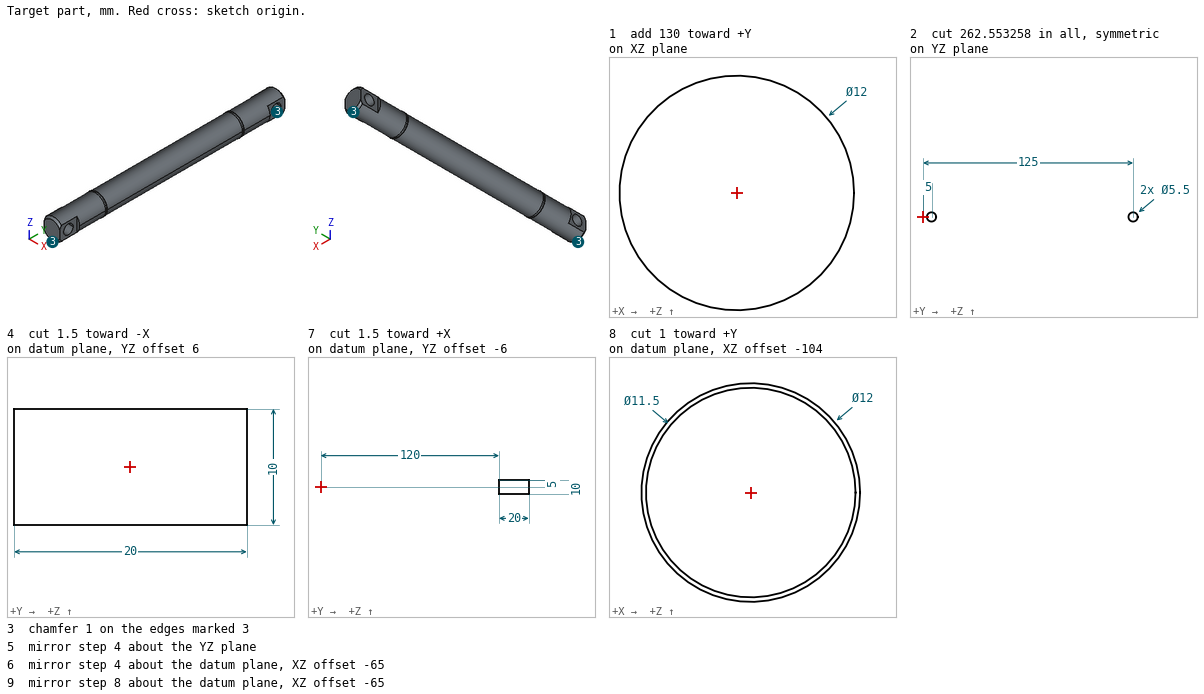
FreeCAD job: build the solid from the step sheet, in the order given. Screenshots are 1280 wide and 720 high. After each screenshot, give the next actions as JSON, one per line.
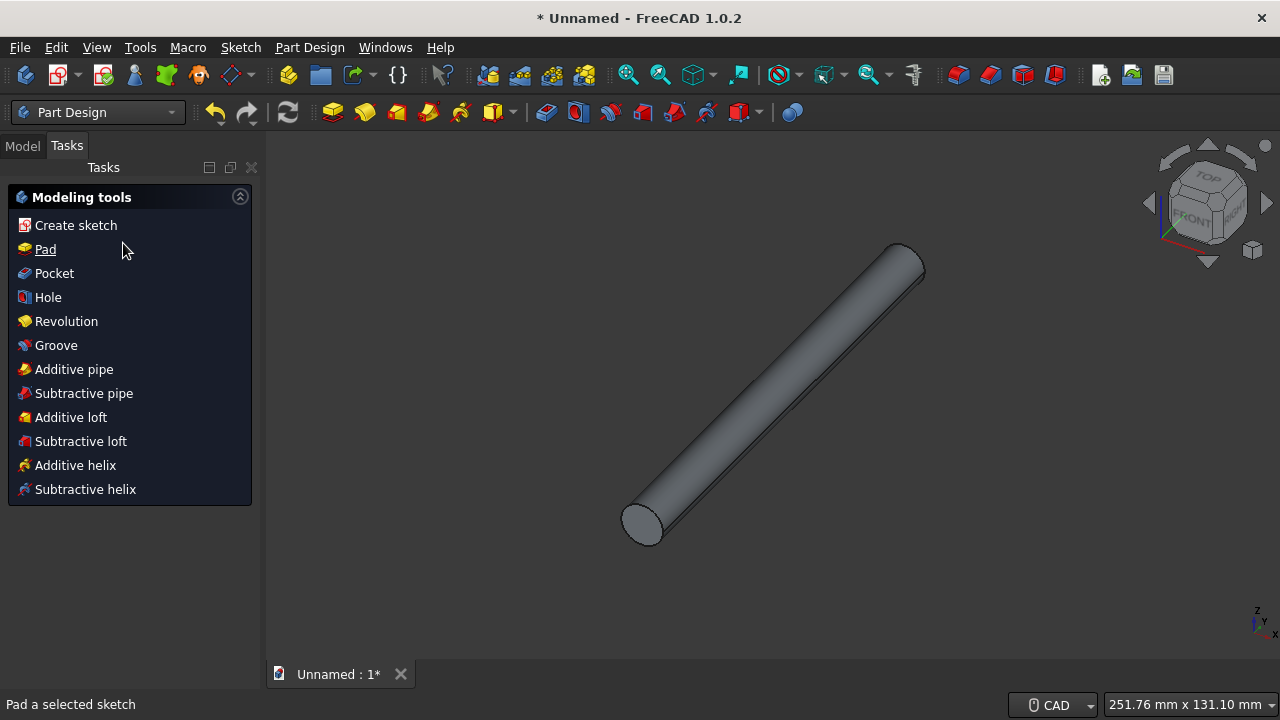
{"action": "left_click", "coordinate": [548, 112]}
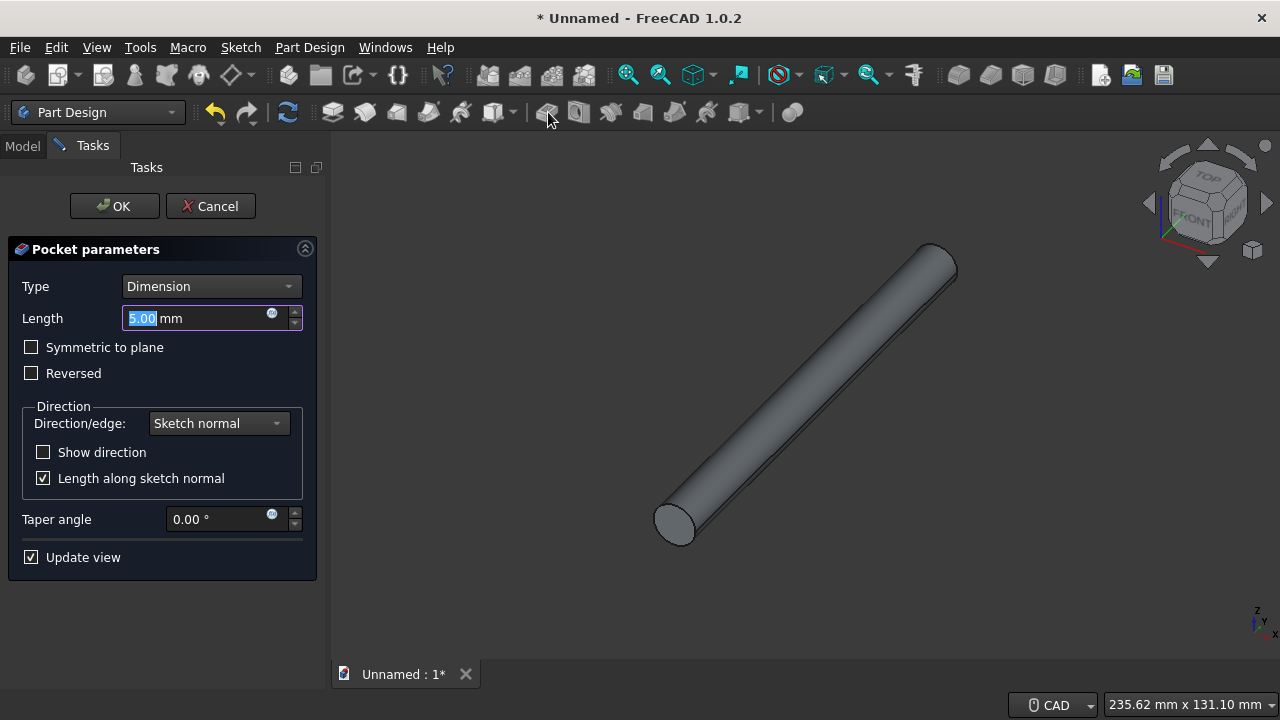
{"action": "type", "text": "262.553258"}
{"action": "key", "text": "Tab"}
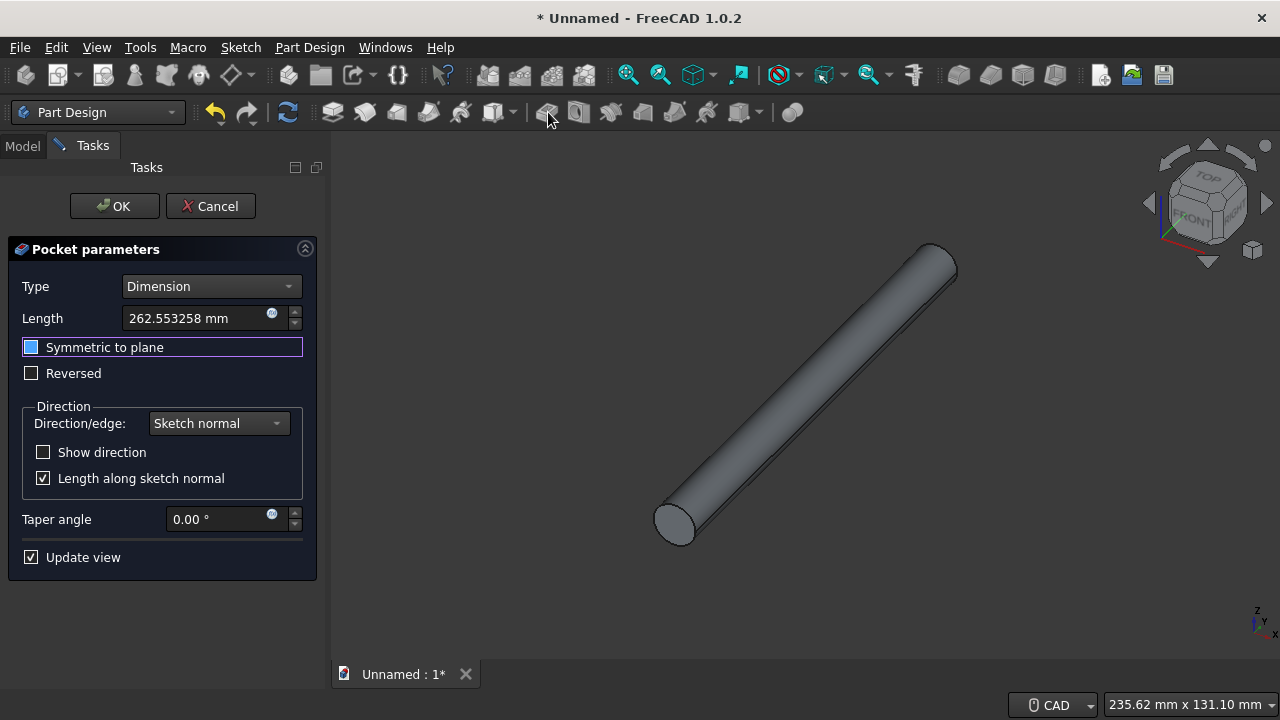
{"action": "left_click", "coordinate": [30, 347]}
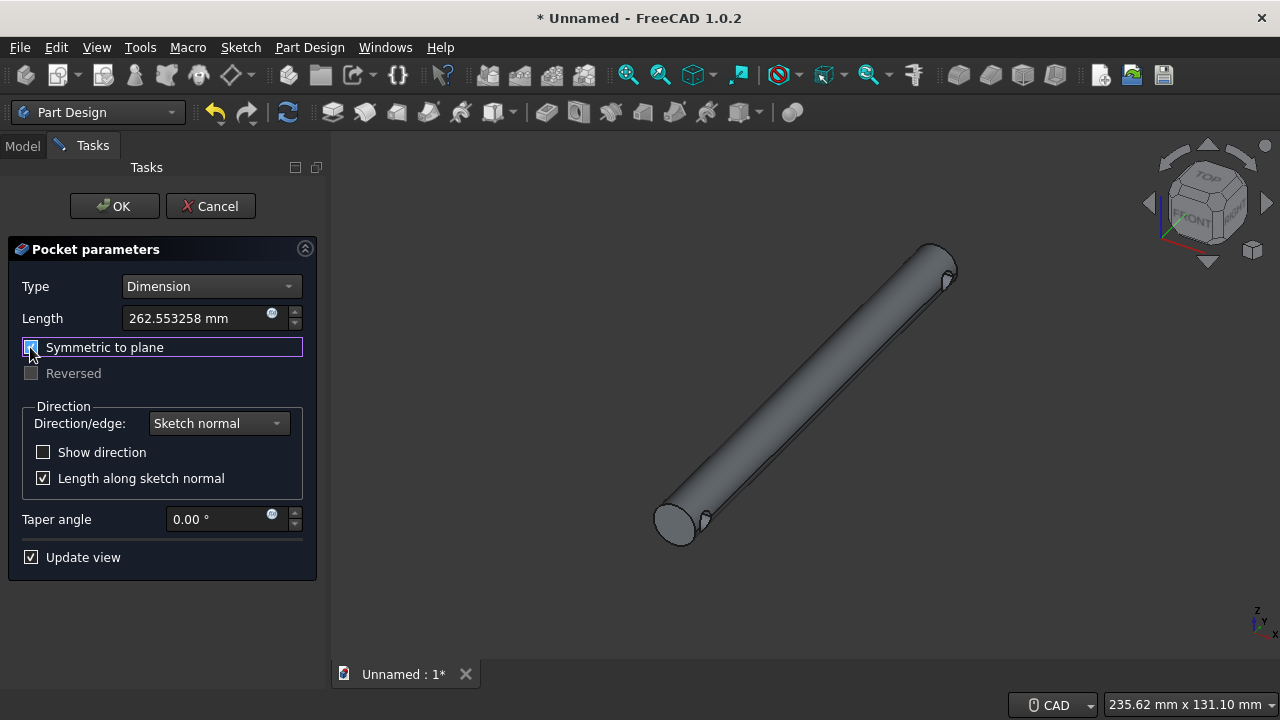
{"action": "left_click", "coordinate": [115, 206]}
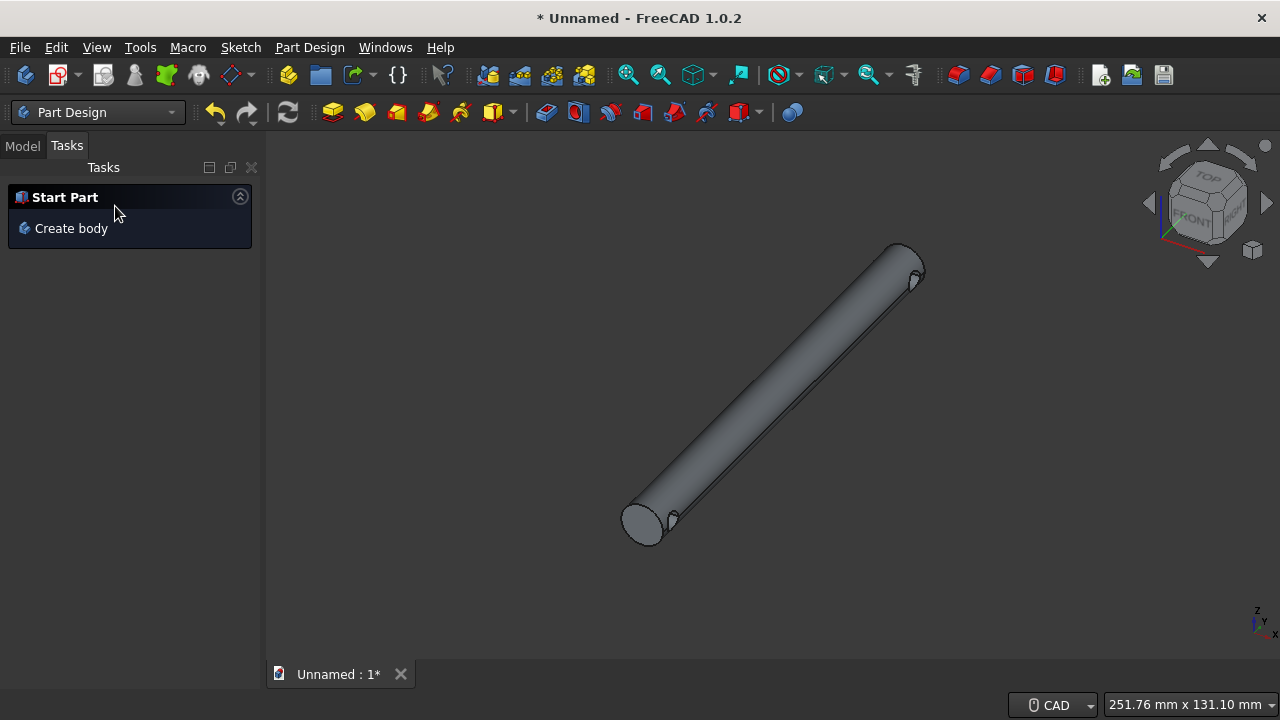
{"action": "left_click", "coordinate": [621, 517]}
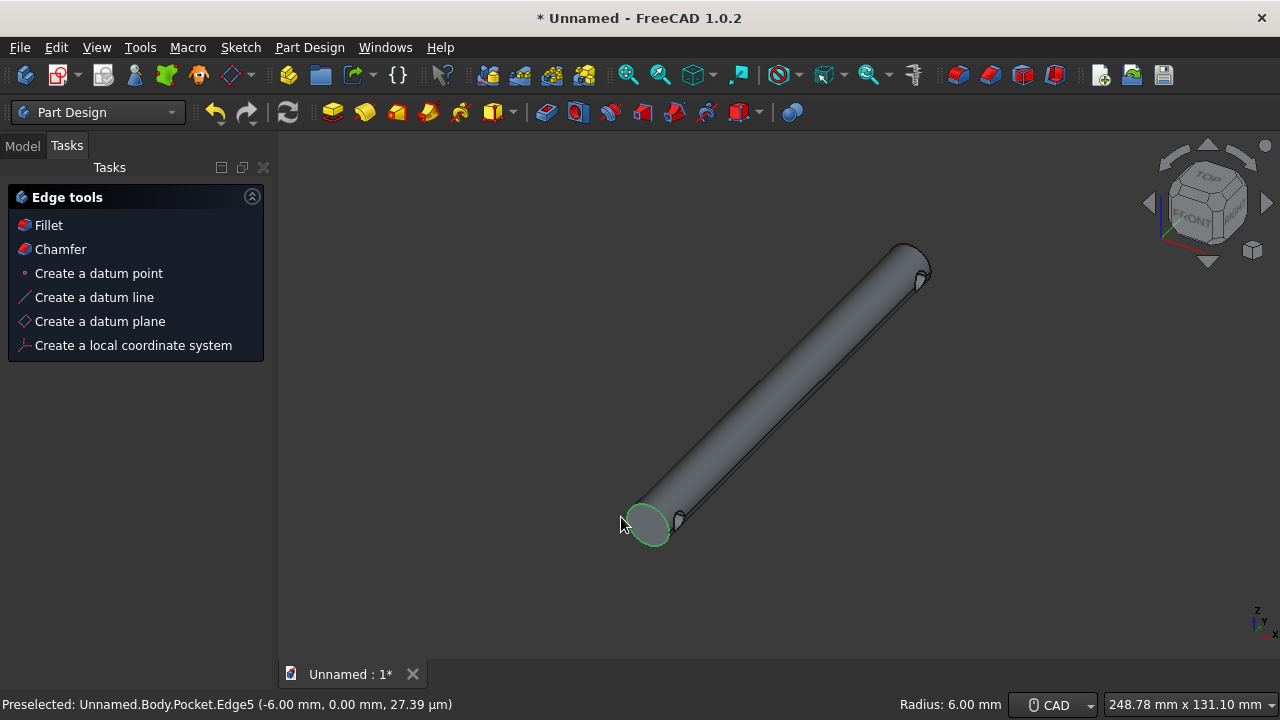
{"action": "key", "text": "0"}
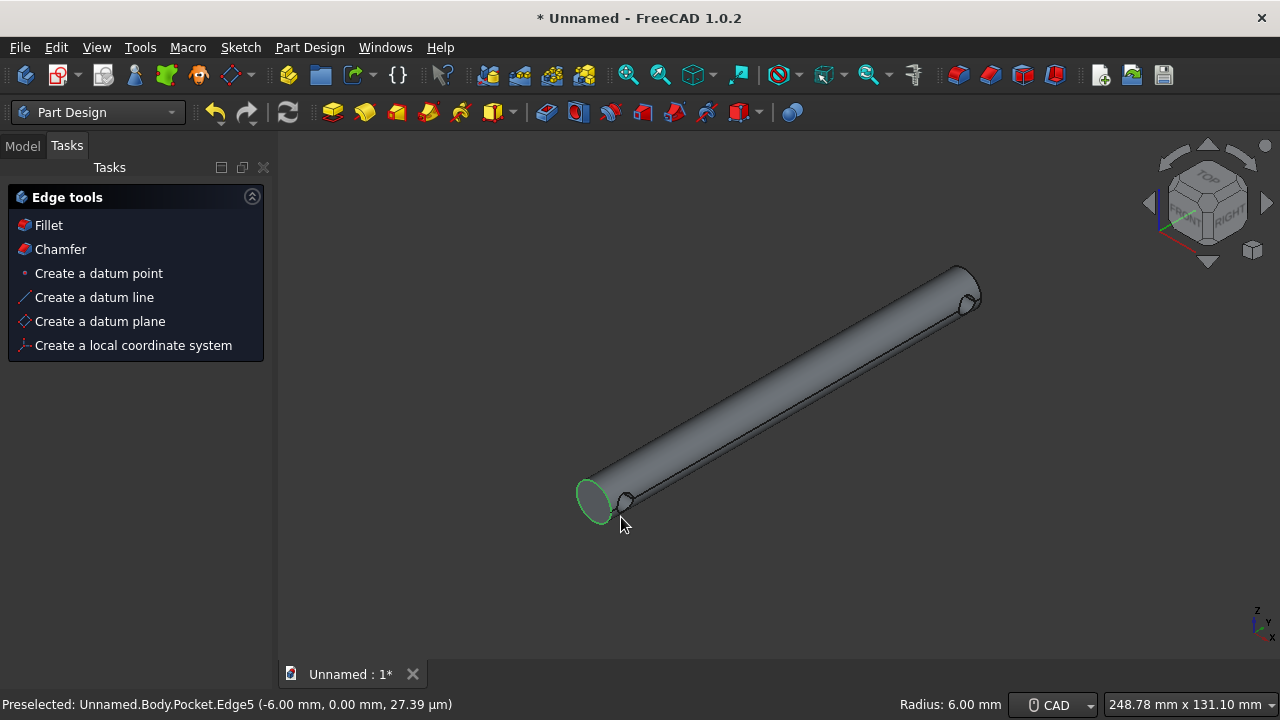
{"action": "left_click", "coordinate": [959, 265], "text": "ctrl"}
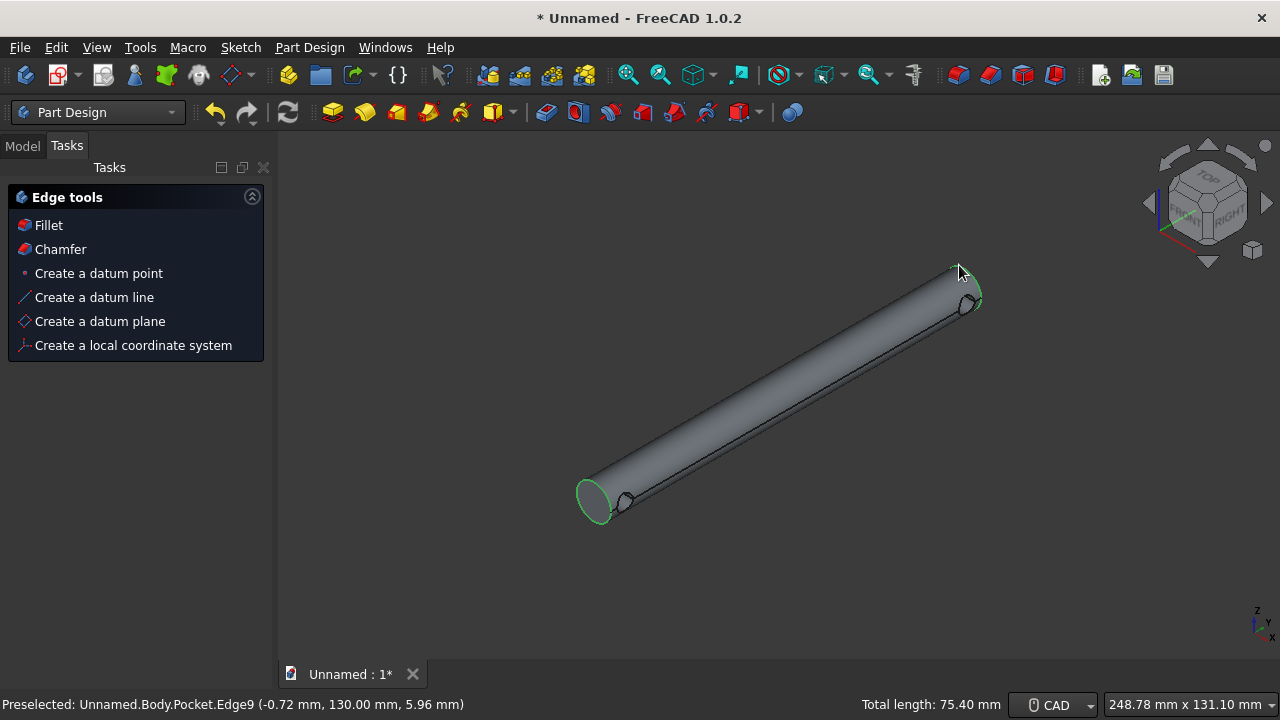
{"action": "left_click", "coordinate": [992, 76]}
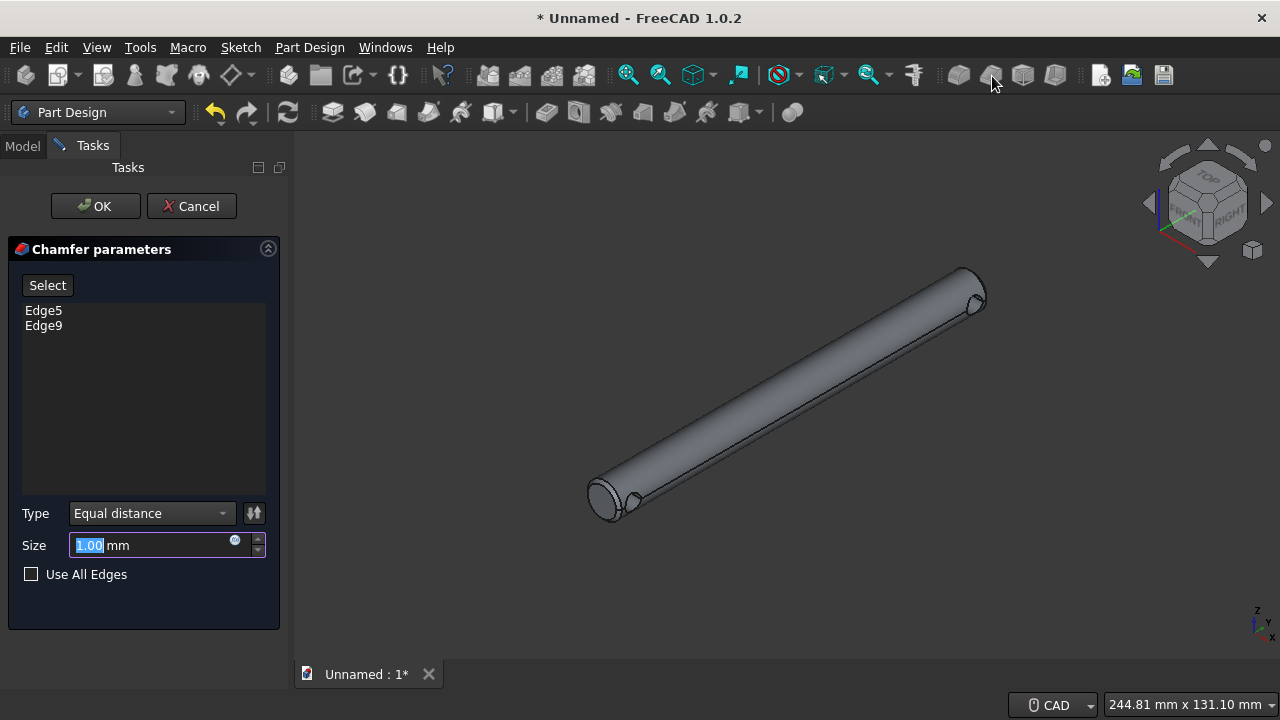
{"action": "type", "text": "1"}
{"action": "key", "text": "Tab"}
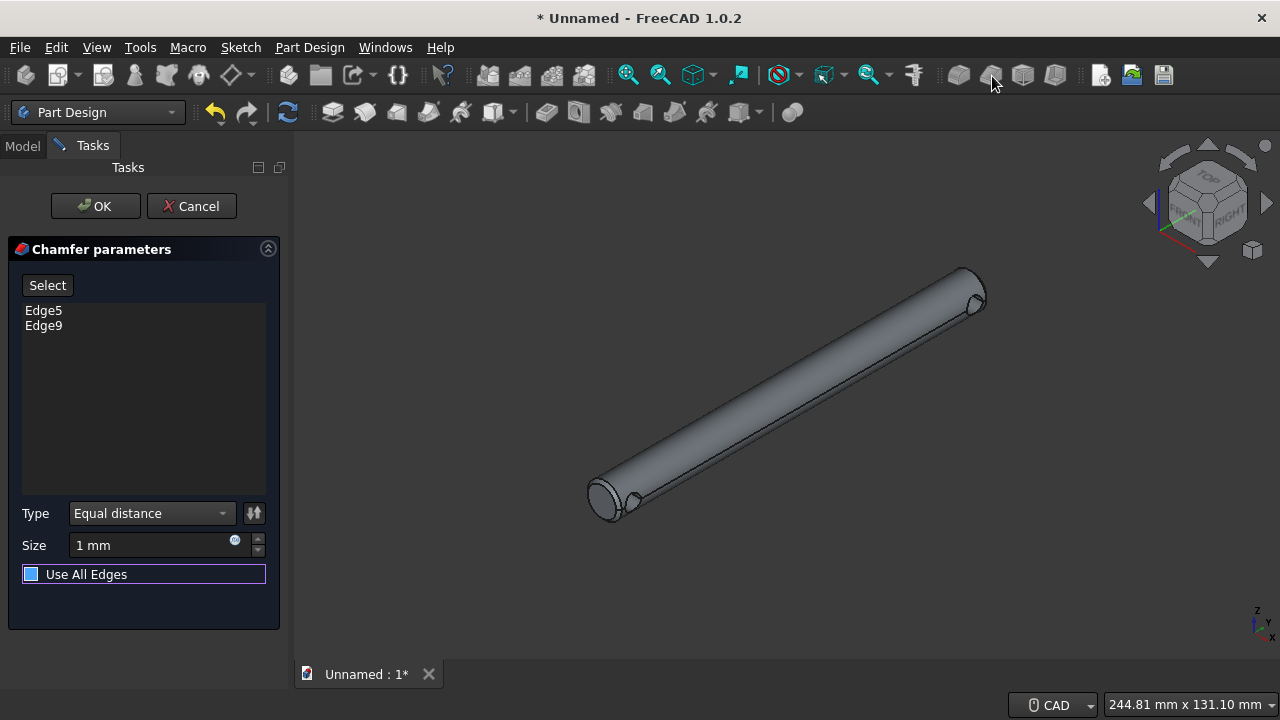
{"action": "left_click", "coordinate": [96, 206]}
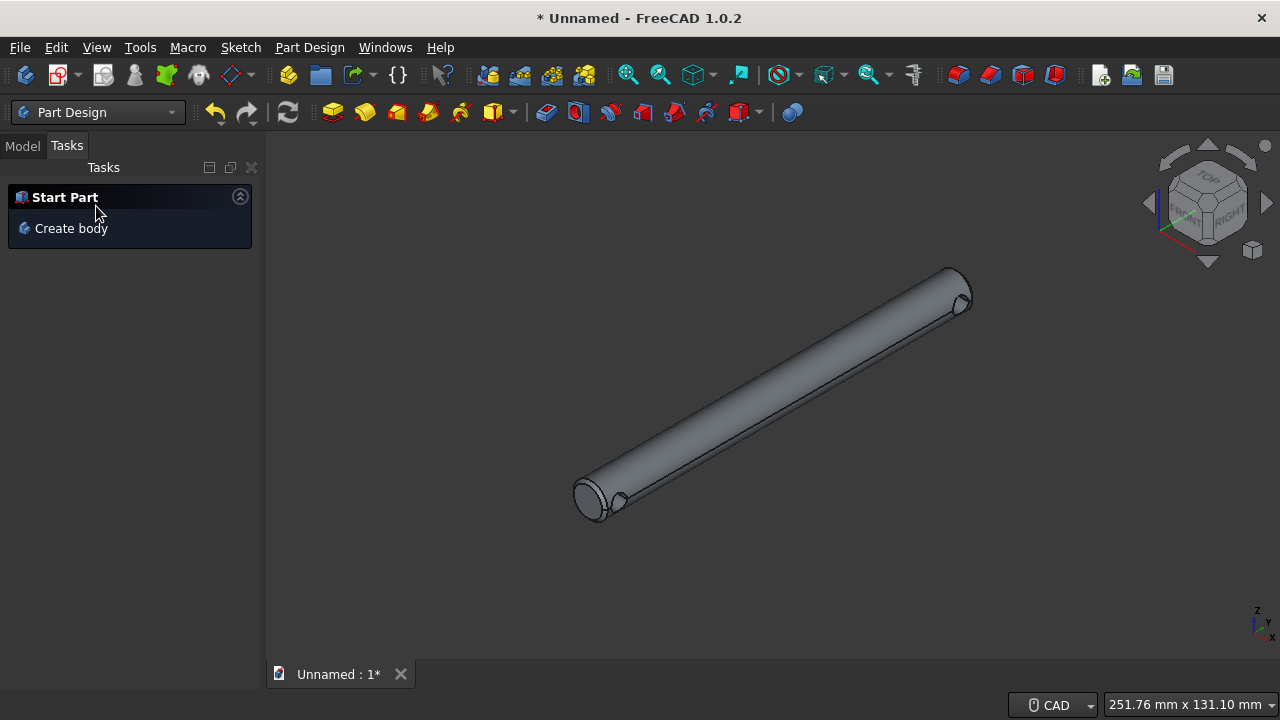
{"action": "left_click", "coordinate": [23, 145]}